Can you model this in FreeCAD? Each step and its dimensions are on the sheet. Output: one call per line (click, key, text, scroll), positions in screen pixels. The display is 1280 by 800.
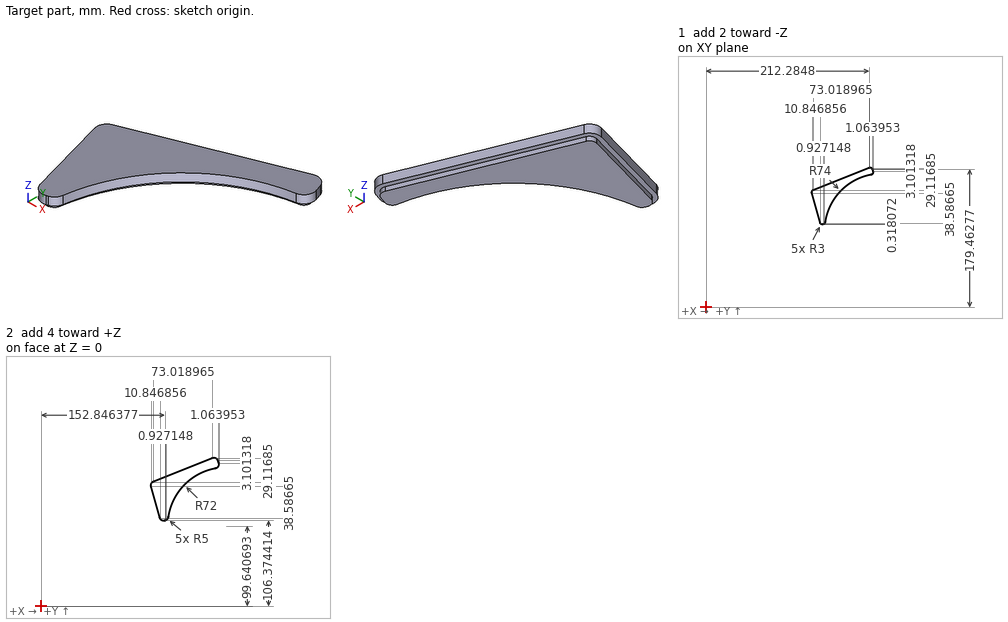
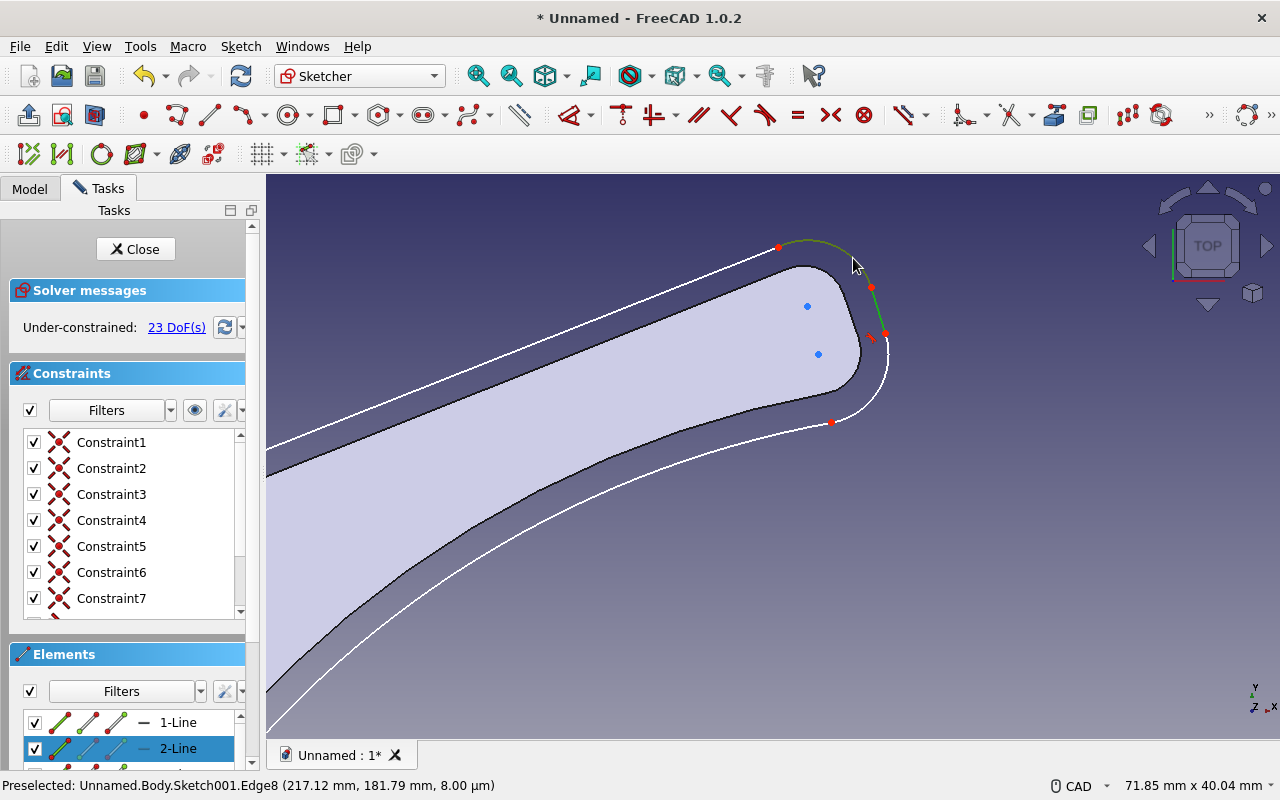
click(765, 116)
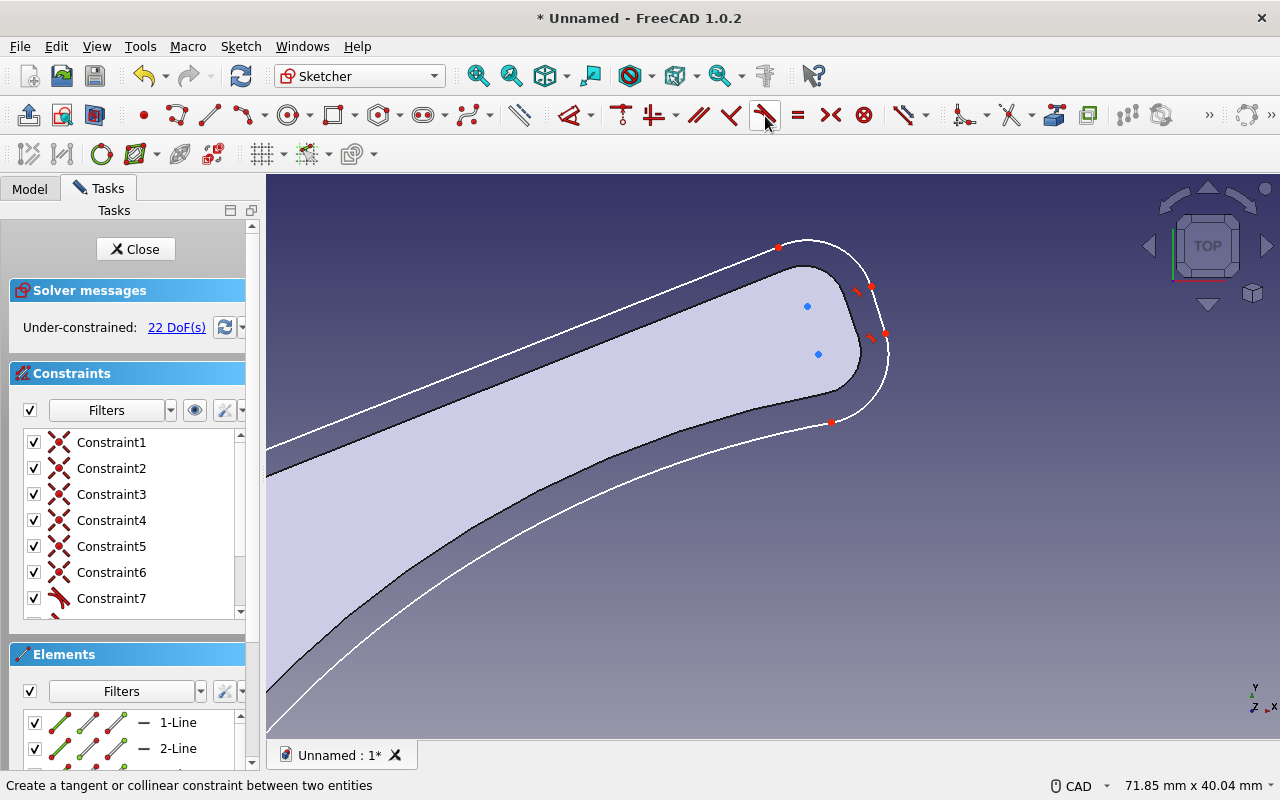
click(468, 370)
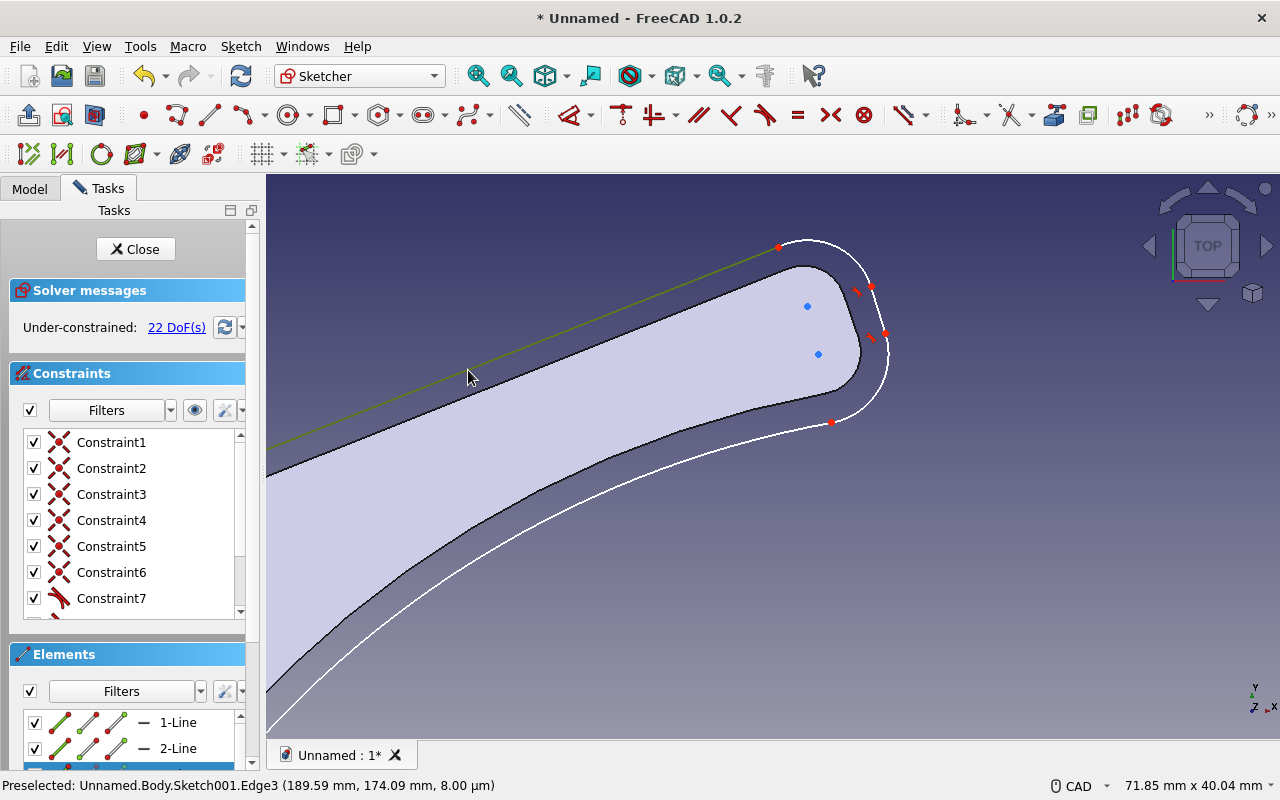
click(853, 258)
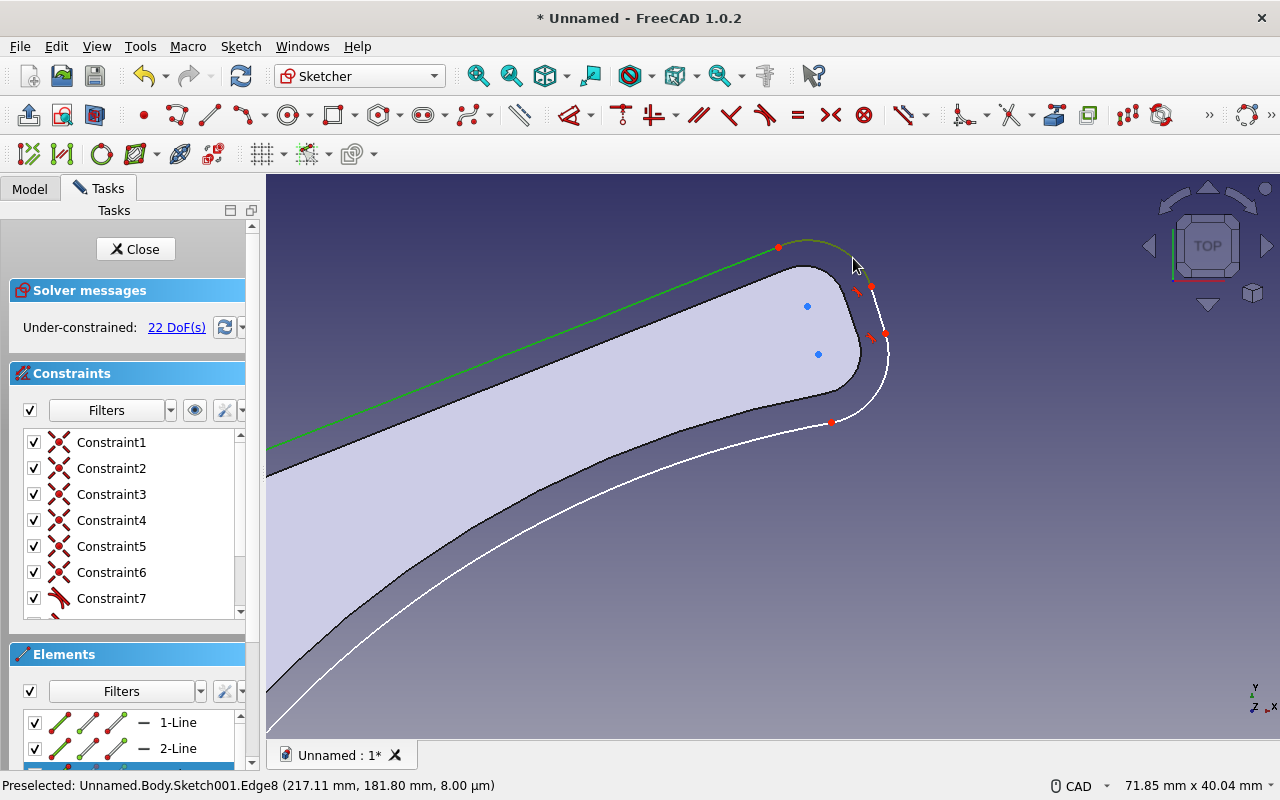
click(765, 116)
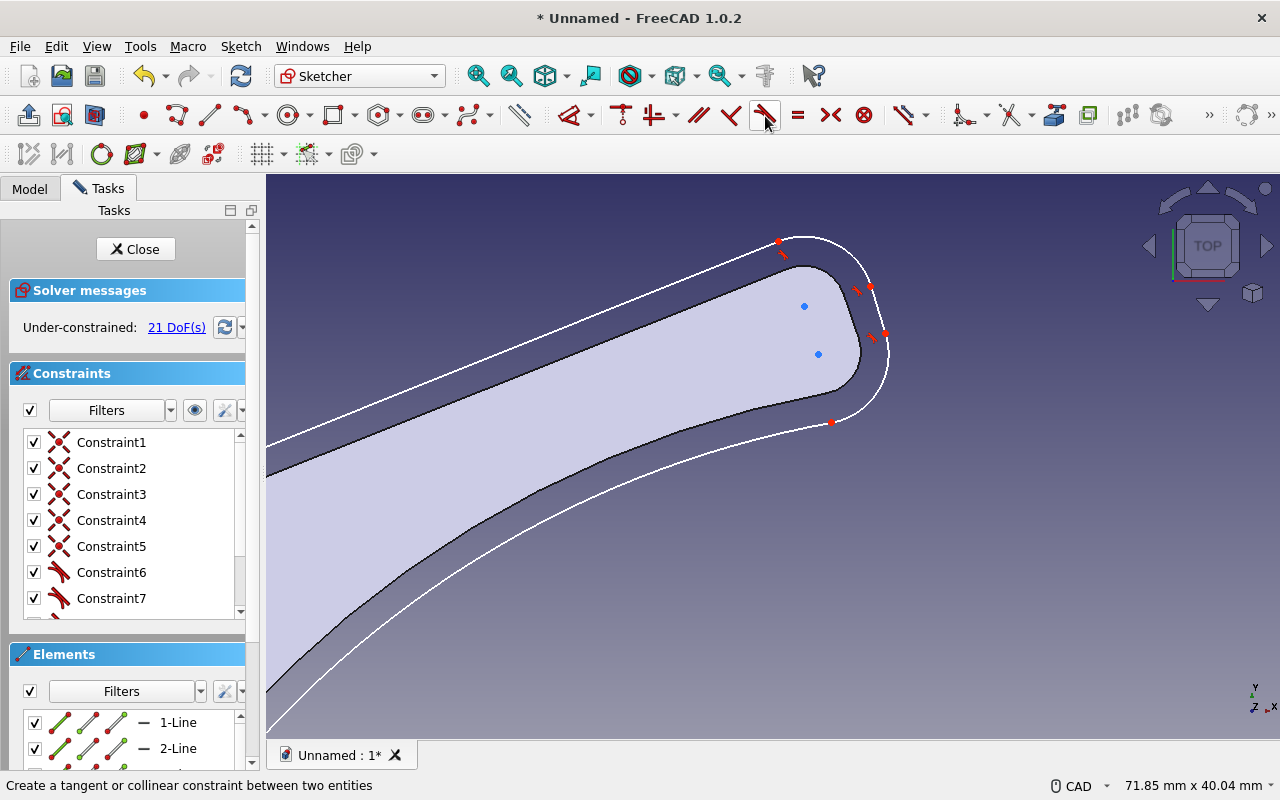
click(468, 366)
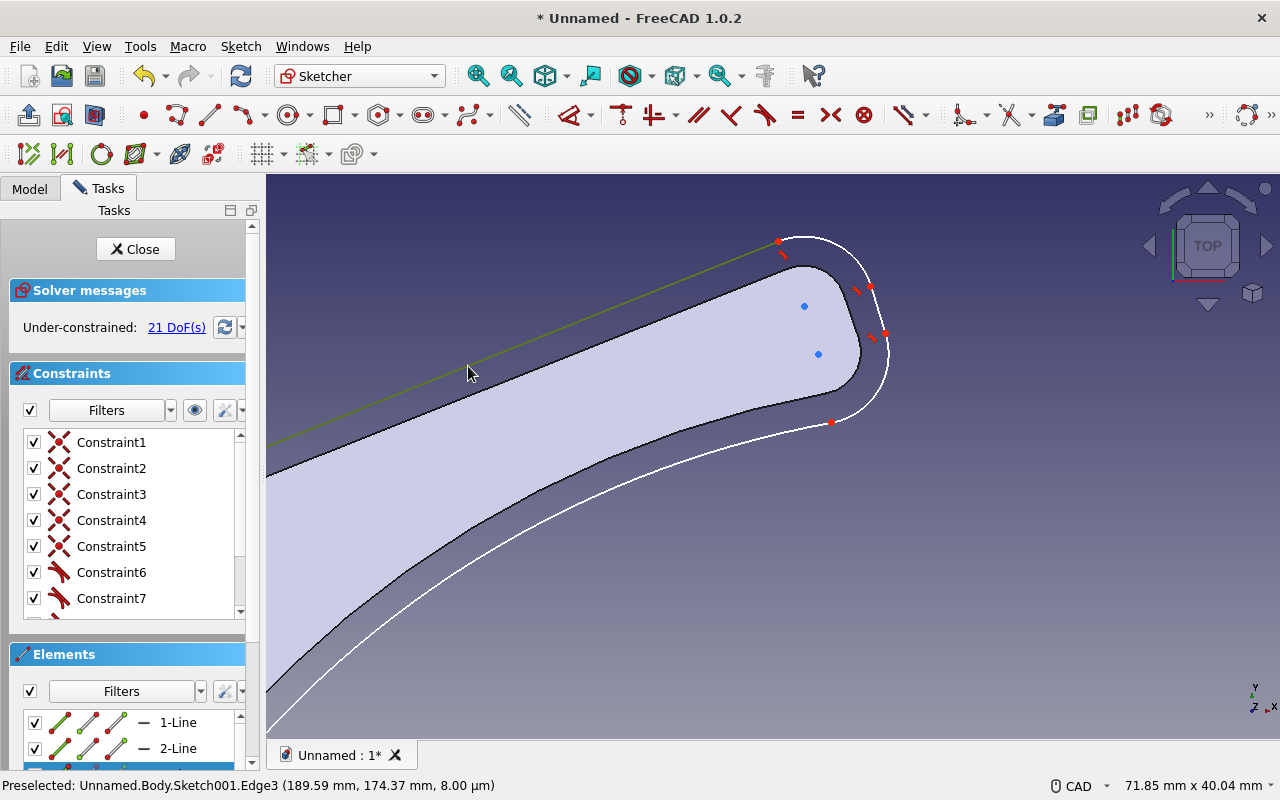
scroll(881, 314, down, 6)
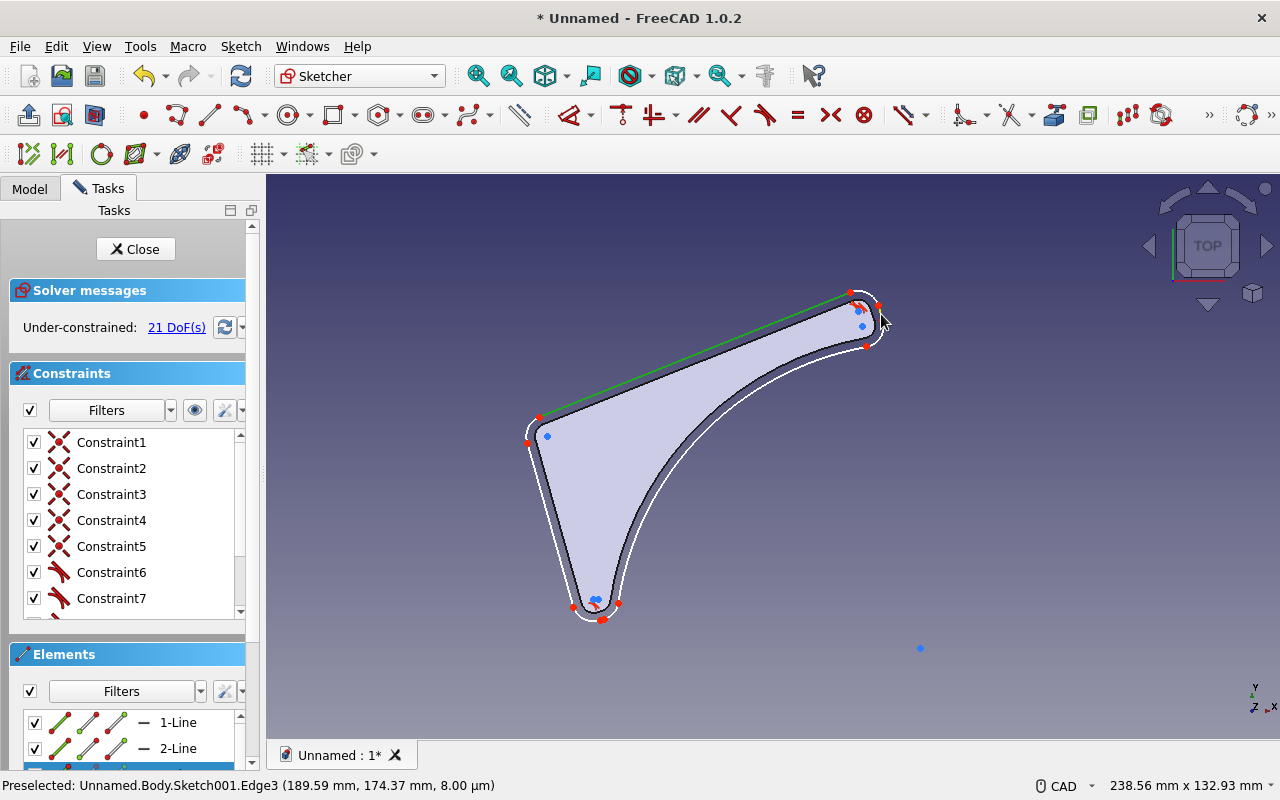
scroll(532, 422, up, 2)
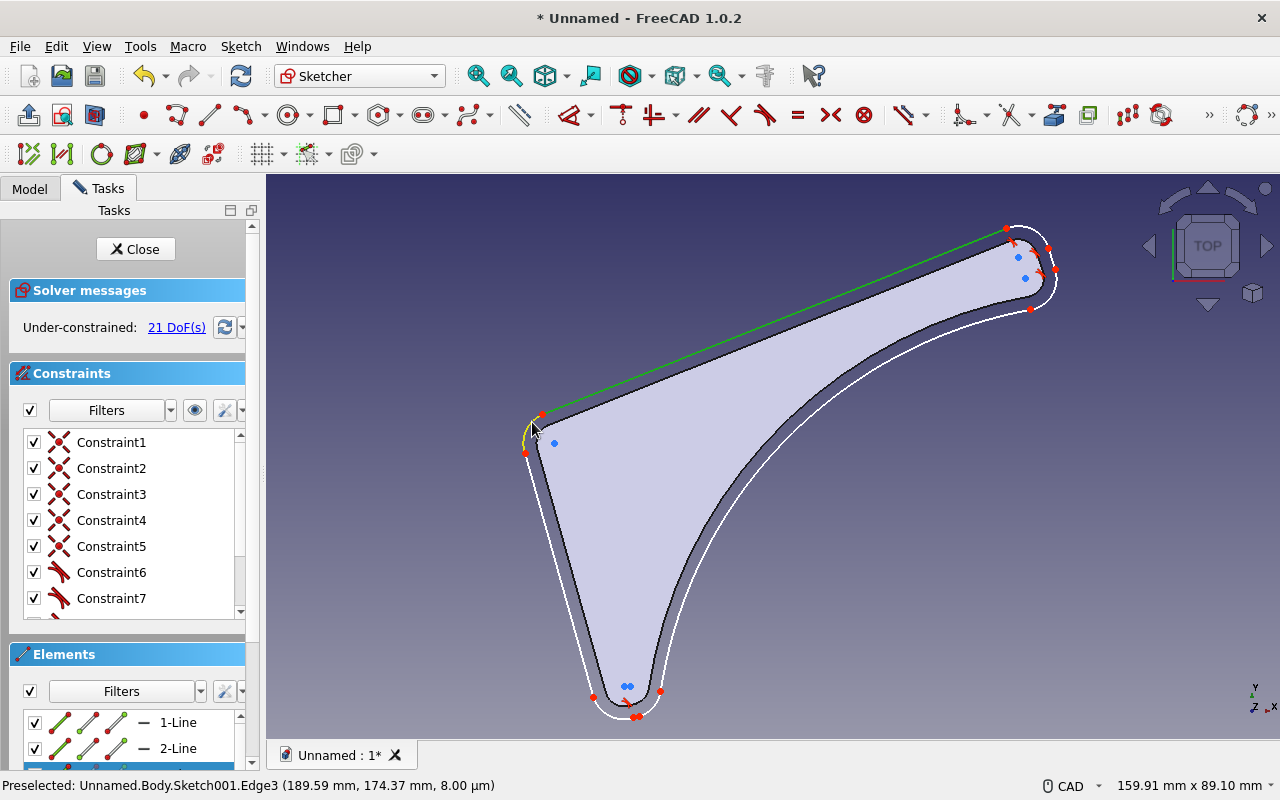
click(531, 422)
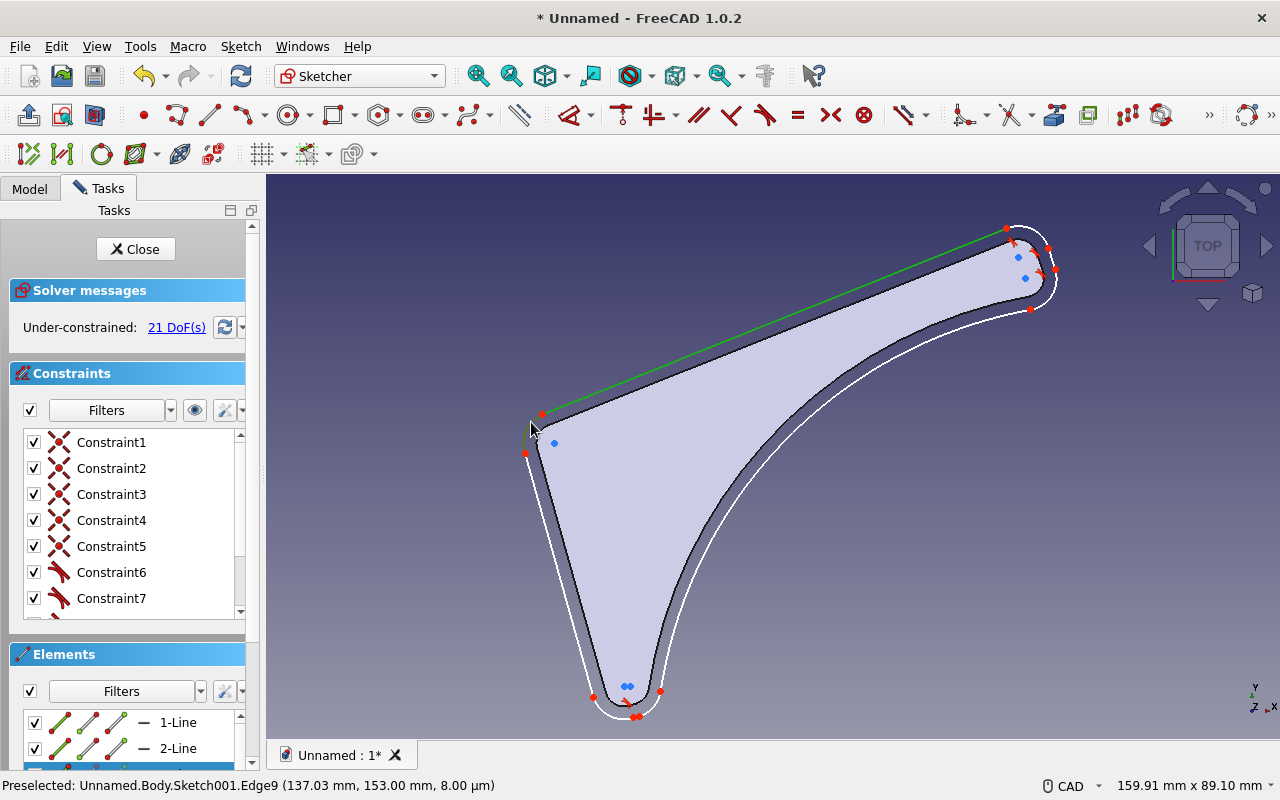
click(765, 116)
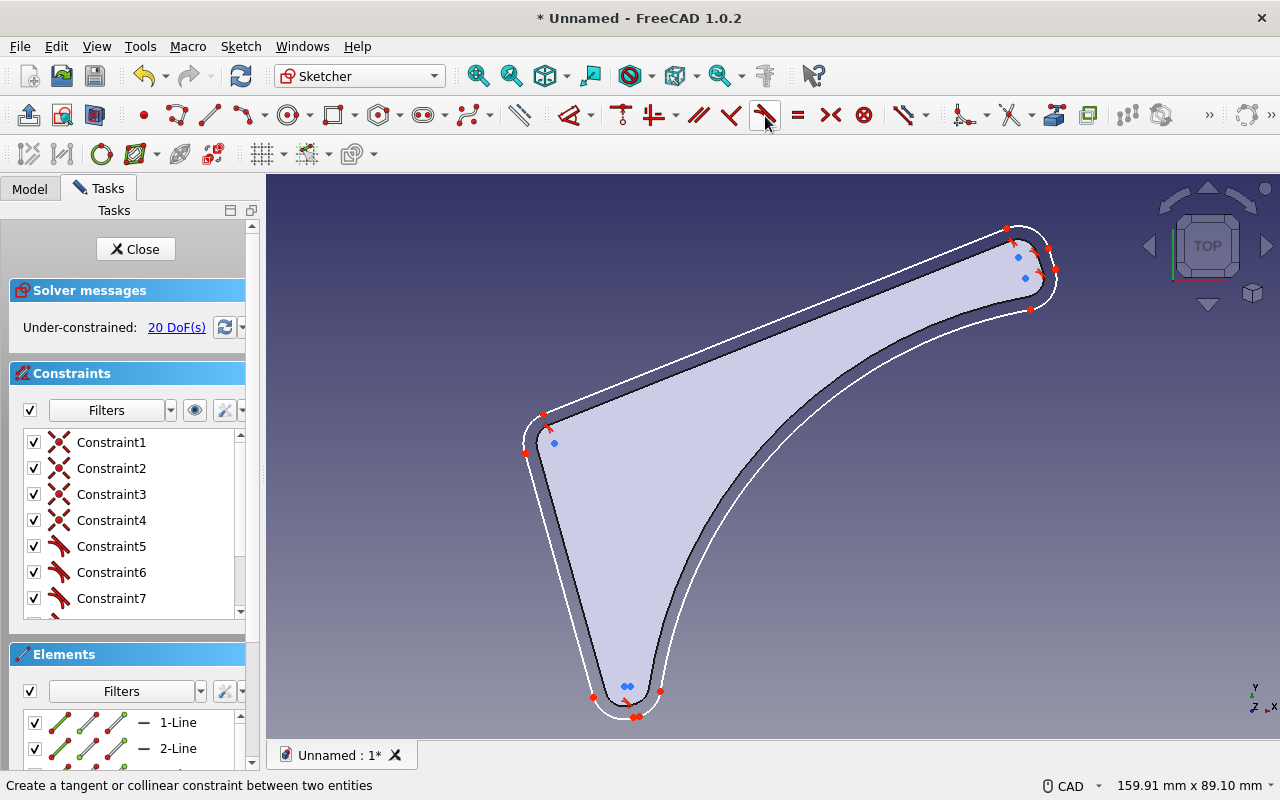
click(546, 527)